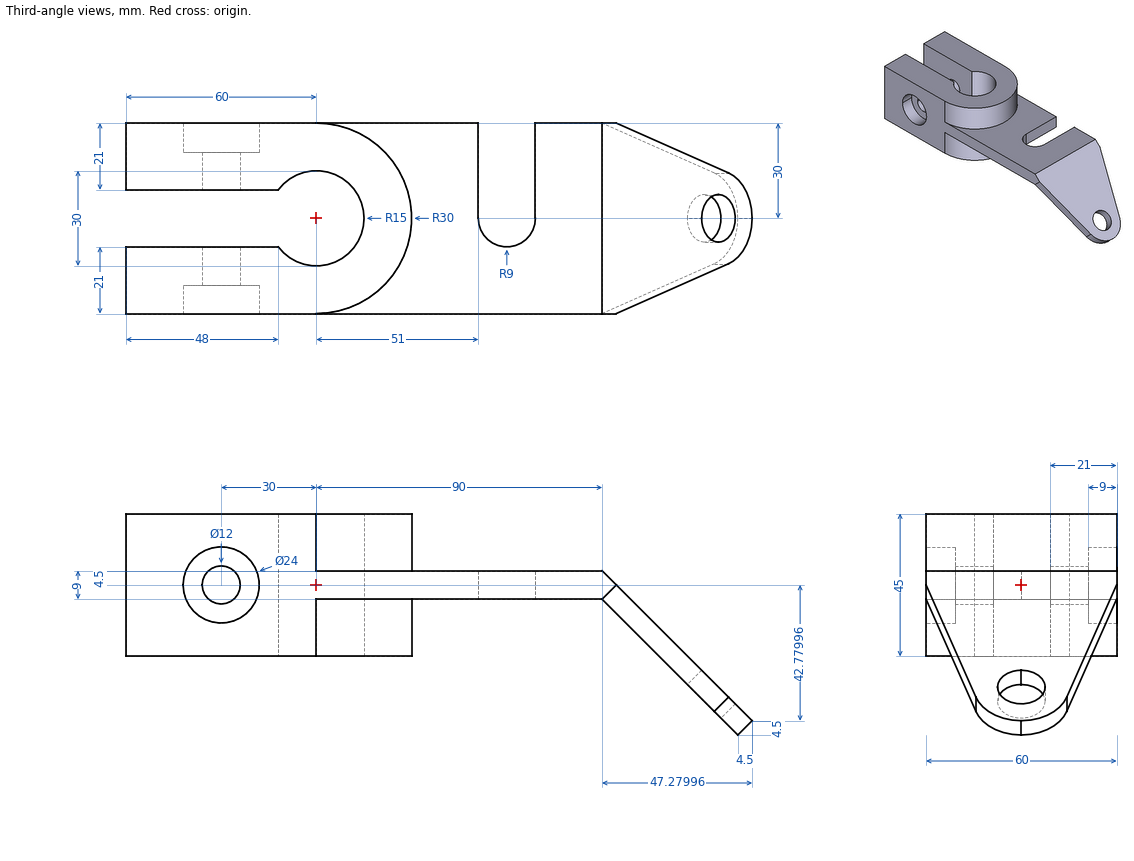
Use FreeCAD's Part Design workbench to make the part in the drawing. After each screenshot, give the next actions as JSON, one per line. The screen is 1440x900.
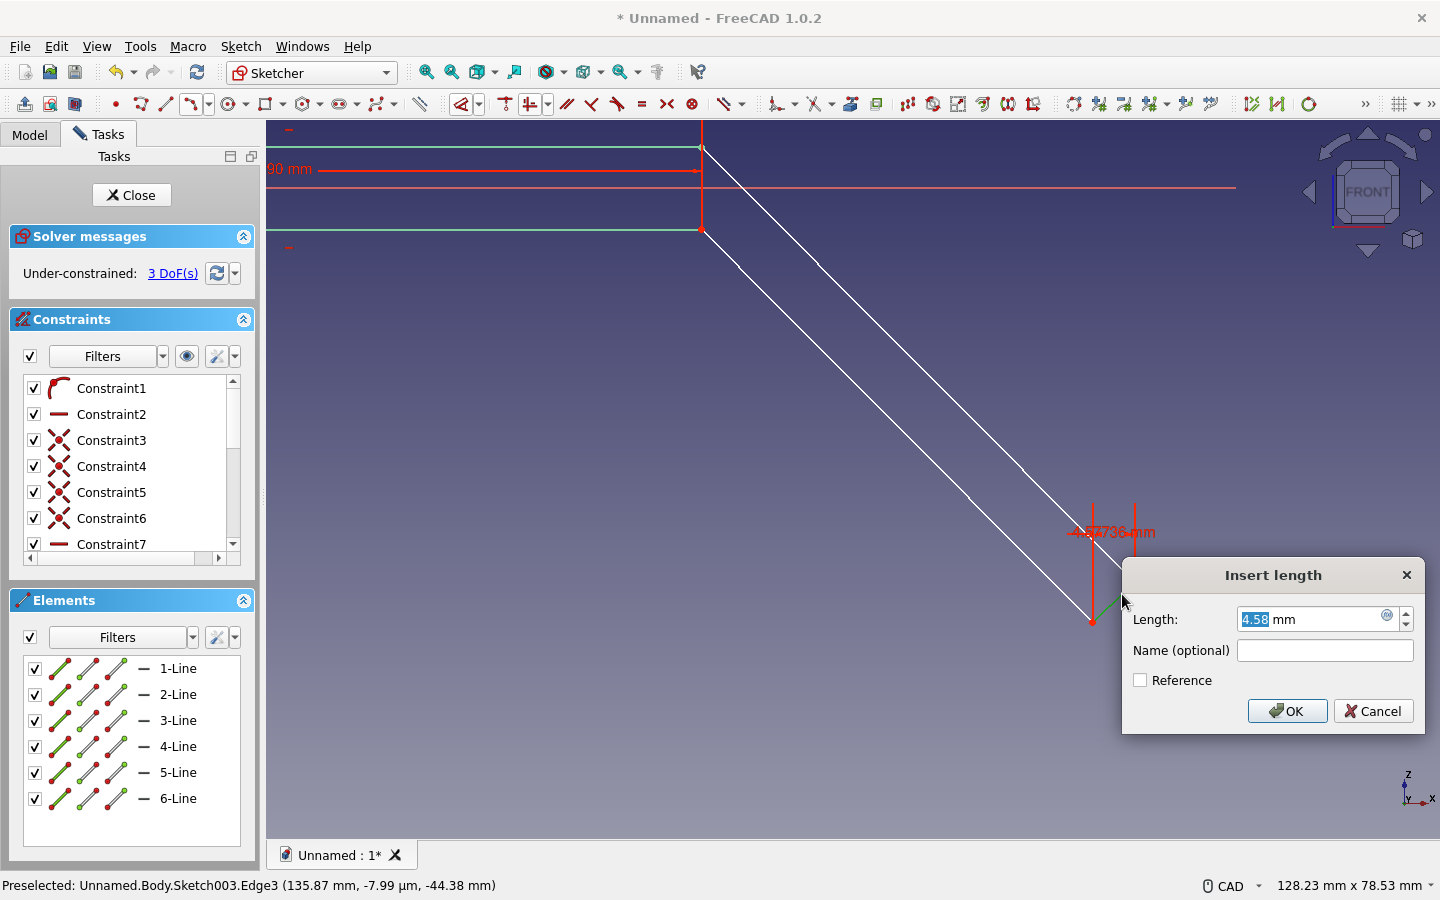
{"action": "type", "text": "4.5"}
{"action": "key", "text": "Return"}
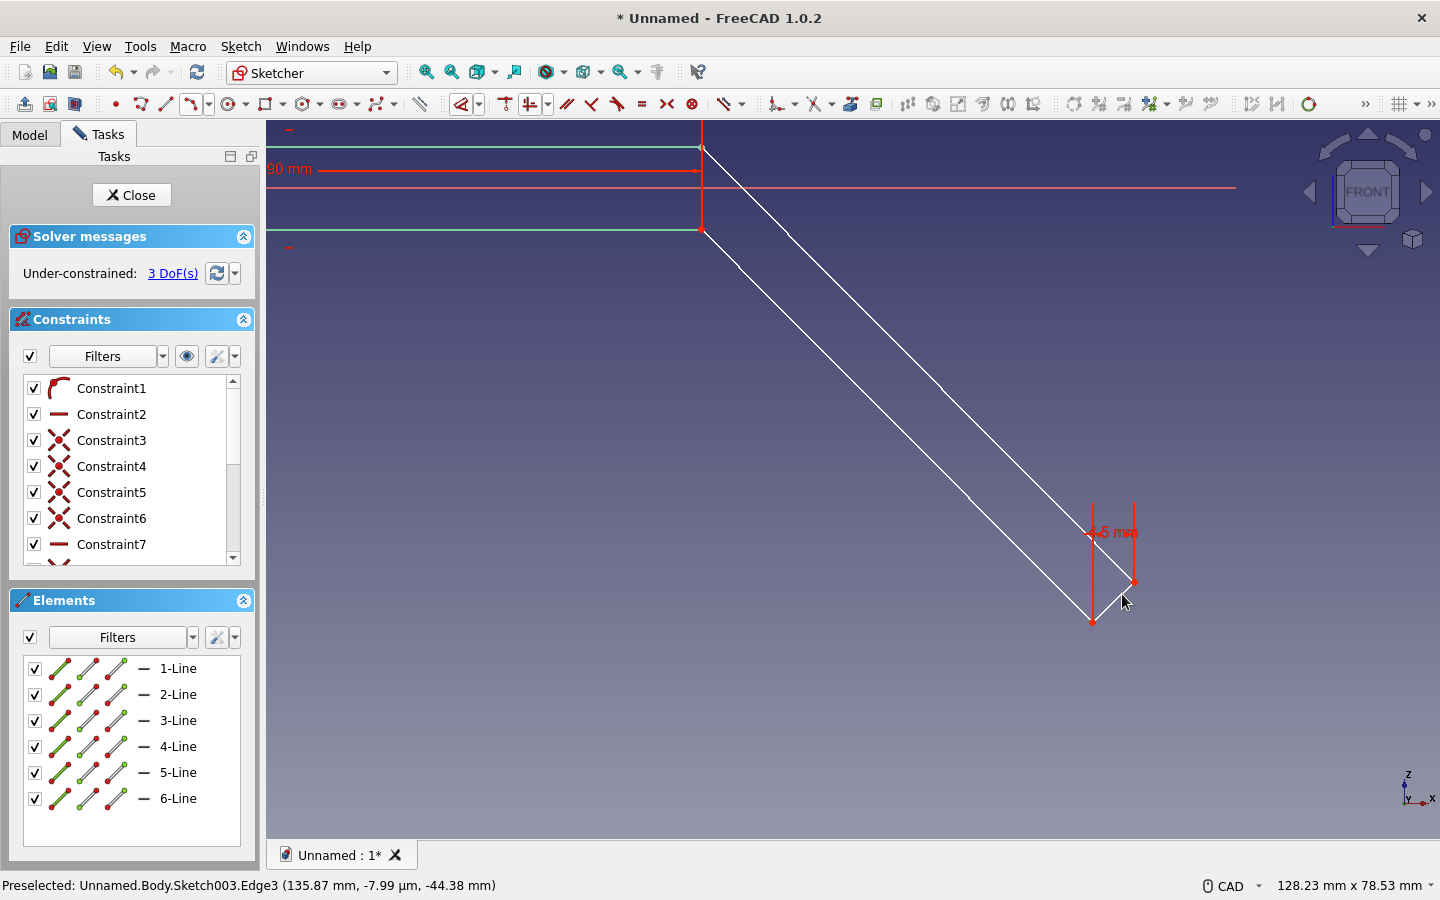
{"action": "left_click", "coordinate": [1122, 594]}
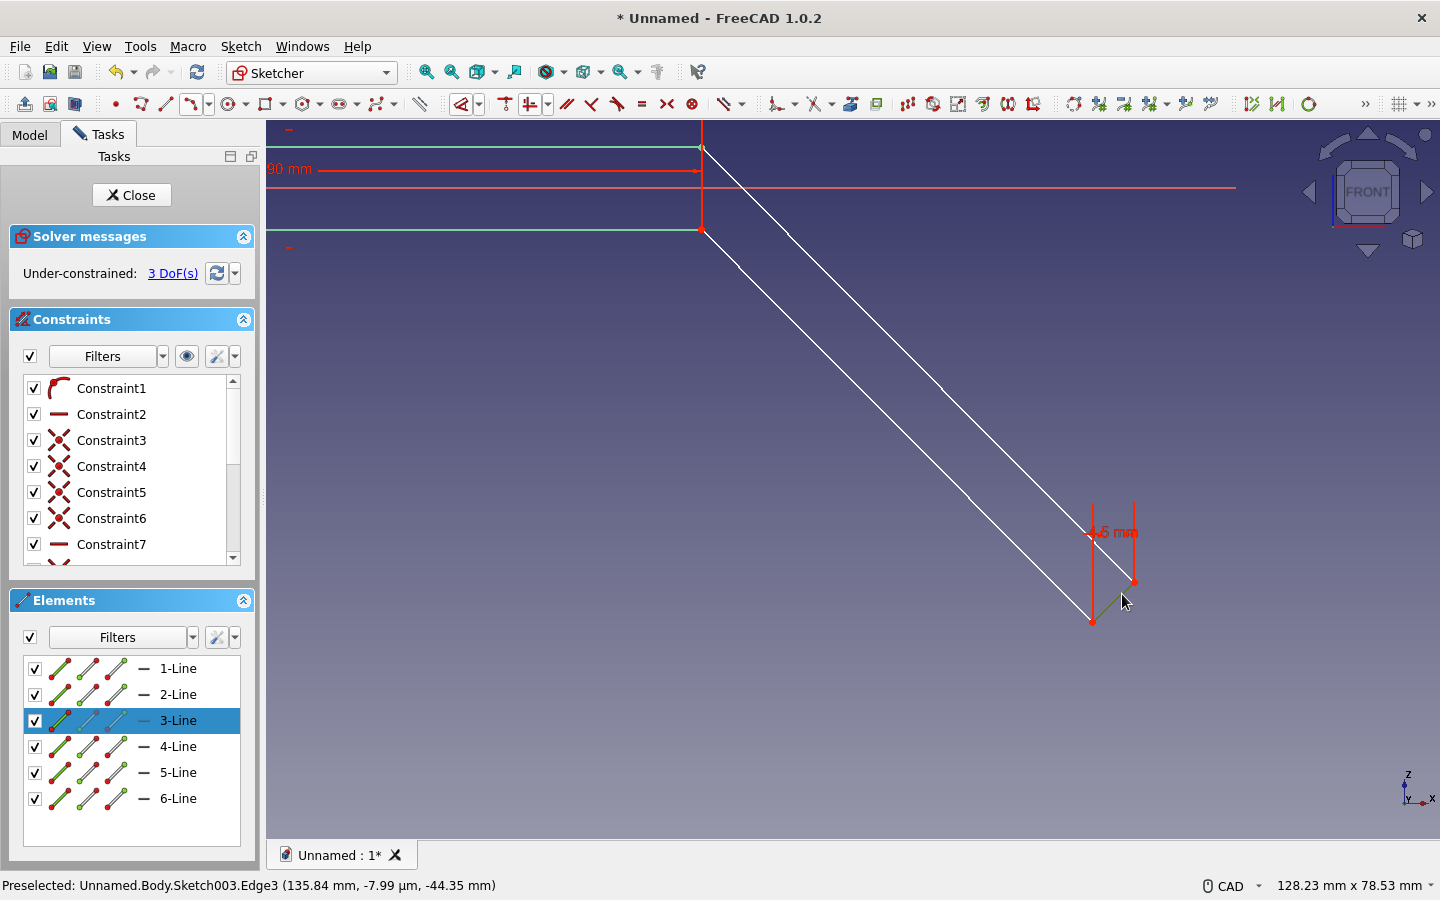
{"action": "key", "text": "i"}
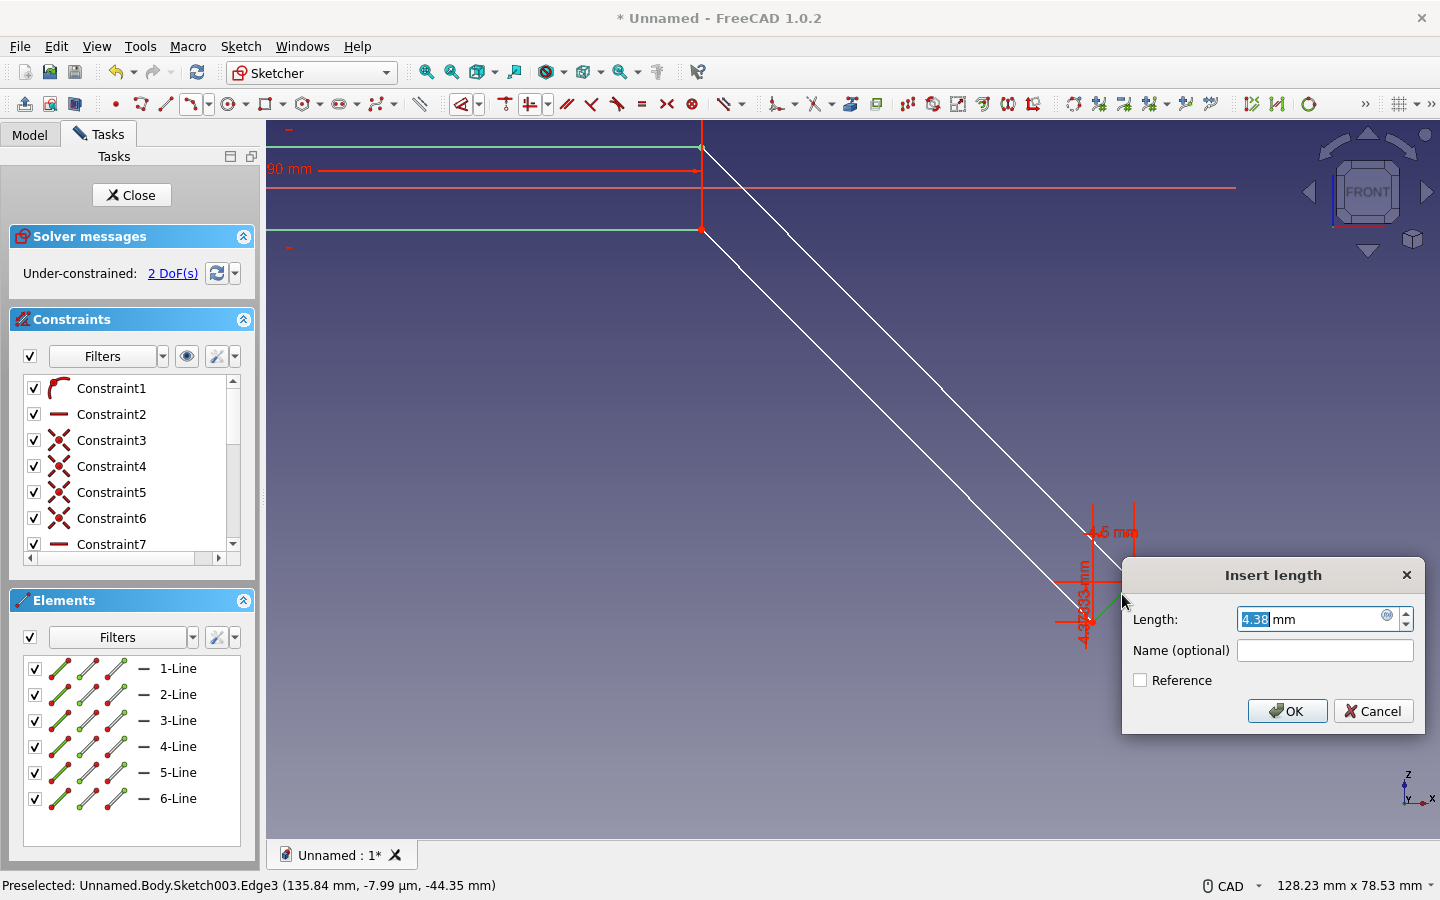
{"action": "type", "text": "4.5"}
{"action": "key", "text": "Return"}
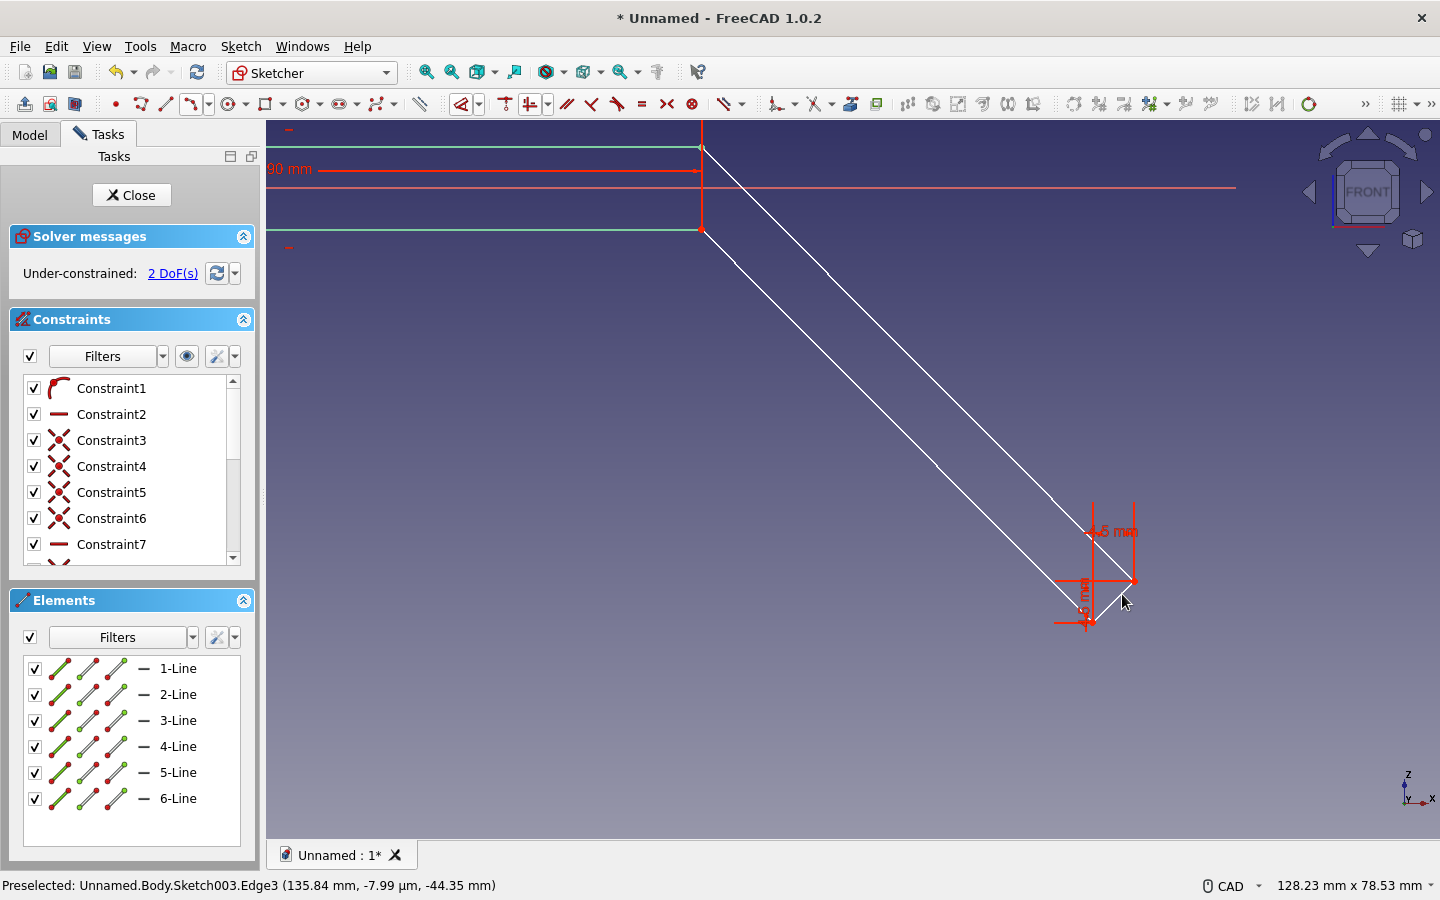
{"action": "left_click", "coordinate": [1134, 581]}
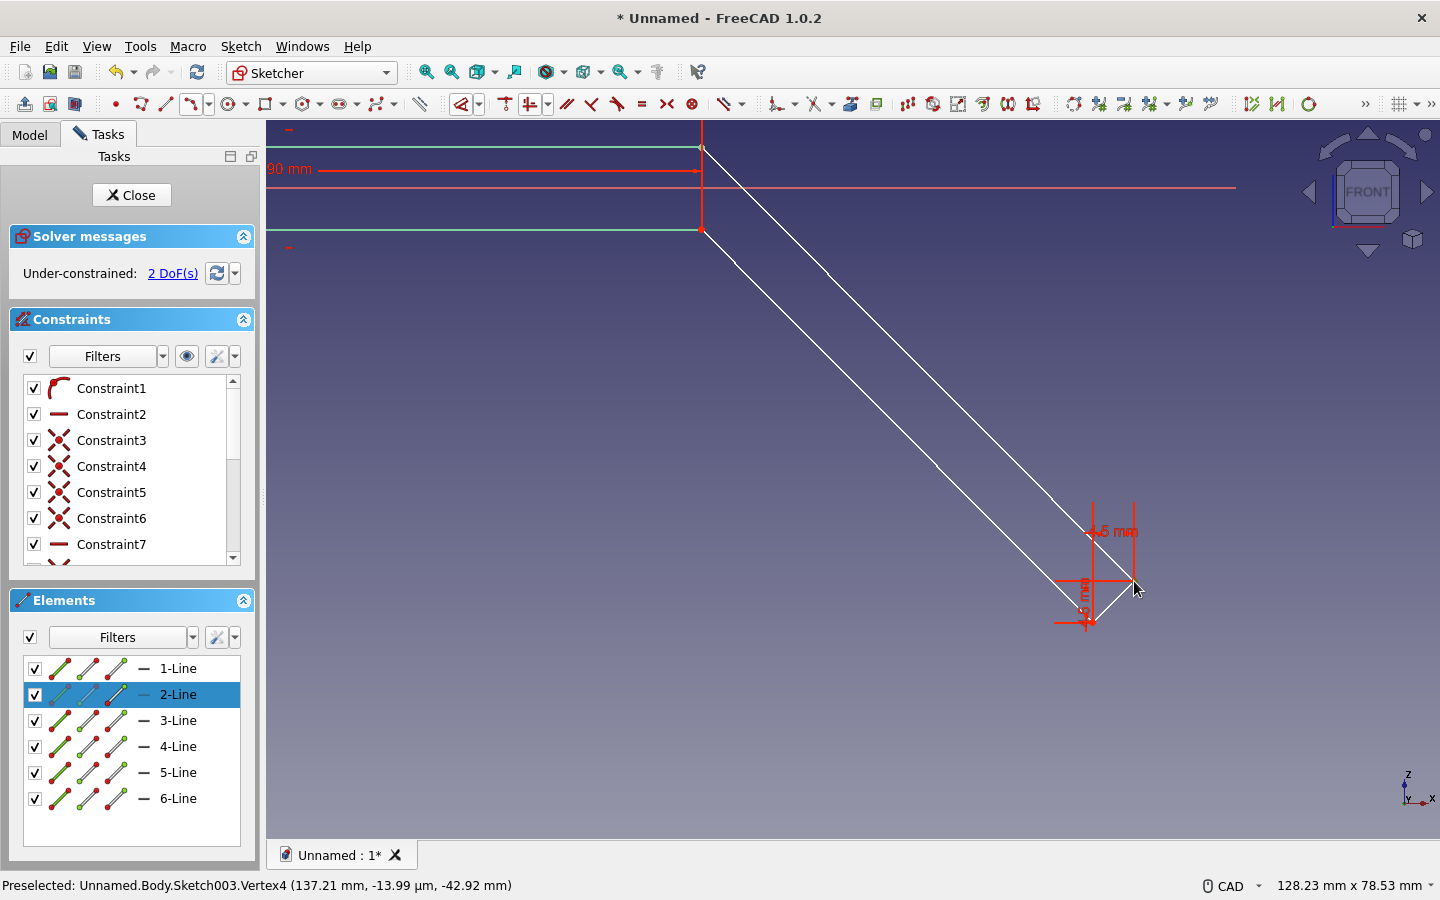
{"action": "key", "text": "i"}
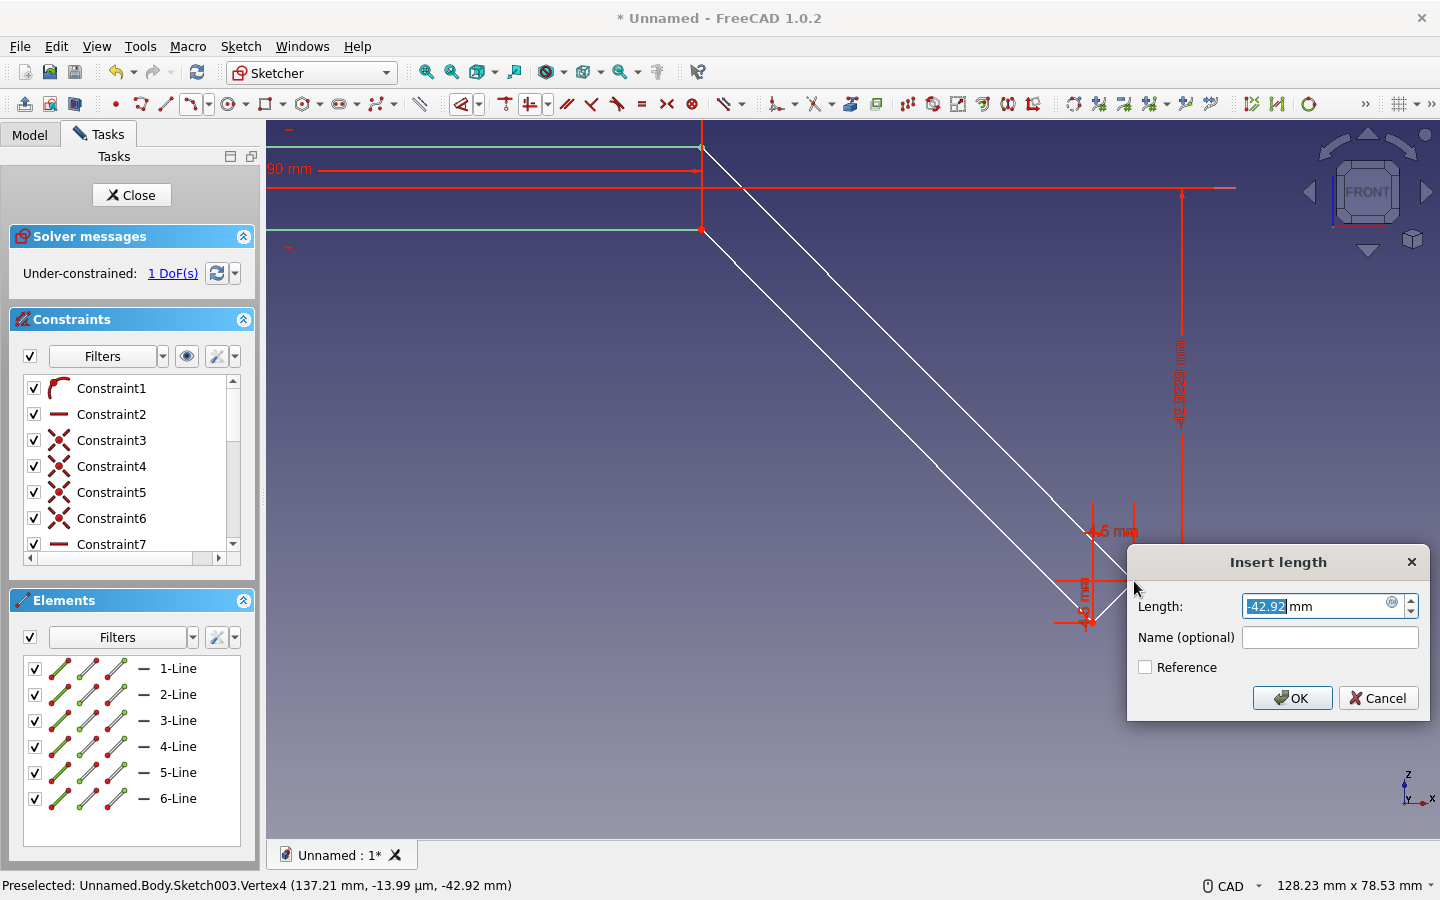
{"action": "type", "text": "-42.77996"}
{"action": "key", "text": "Return"}